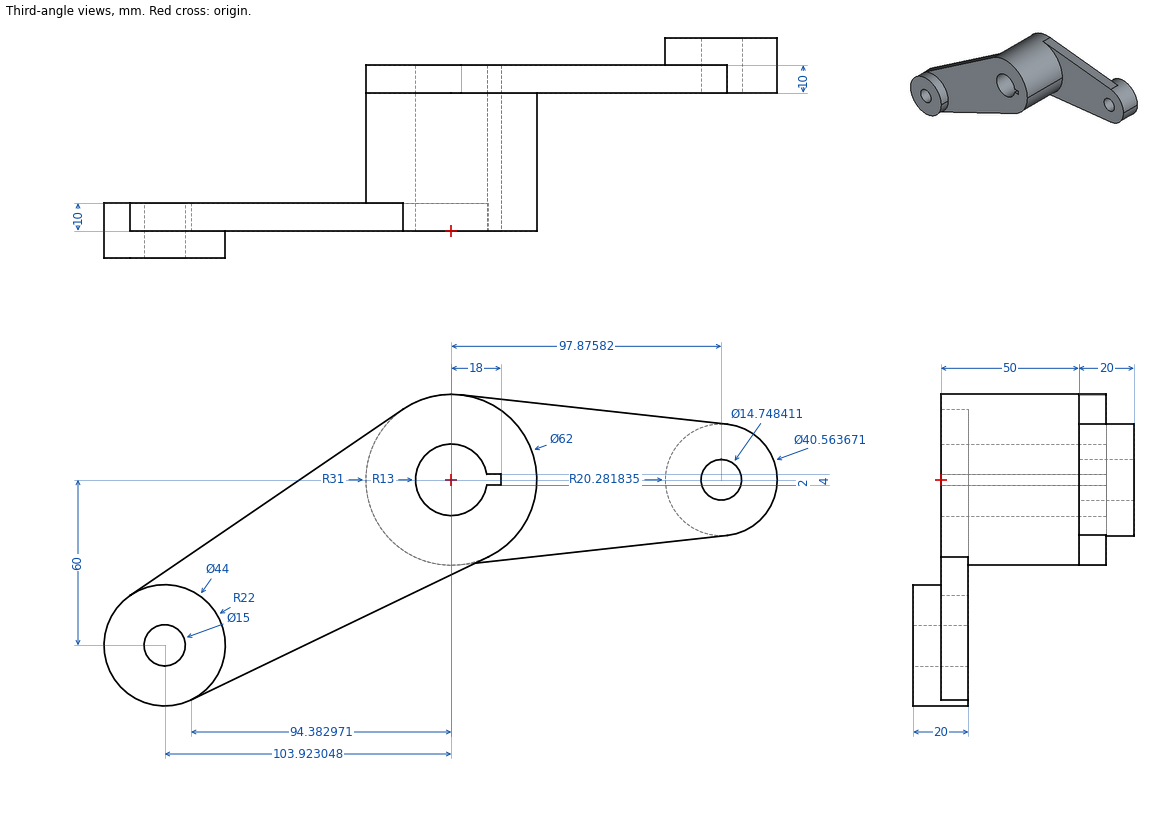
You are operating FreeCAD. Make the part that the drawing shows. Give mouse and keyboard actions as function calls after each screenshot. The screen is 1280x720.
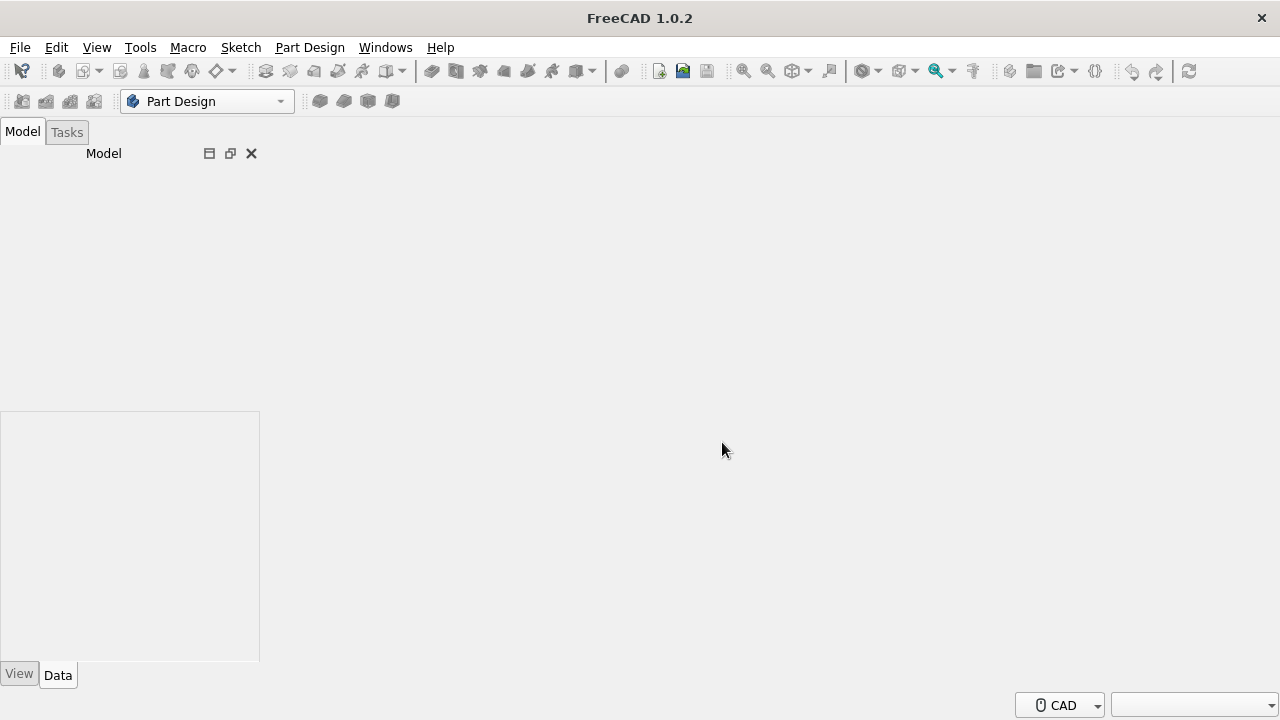
key(ctrl+n)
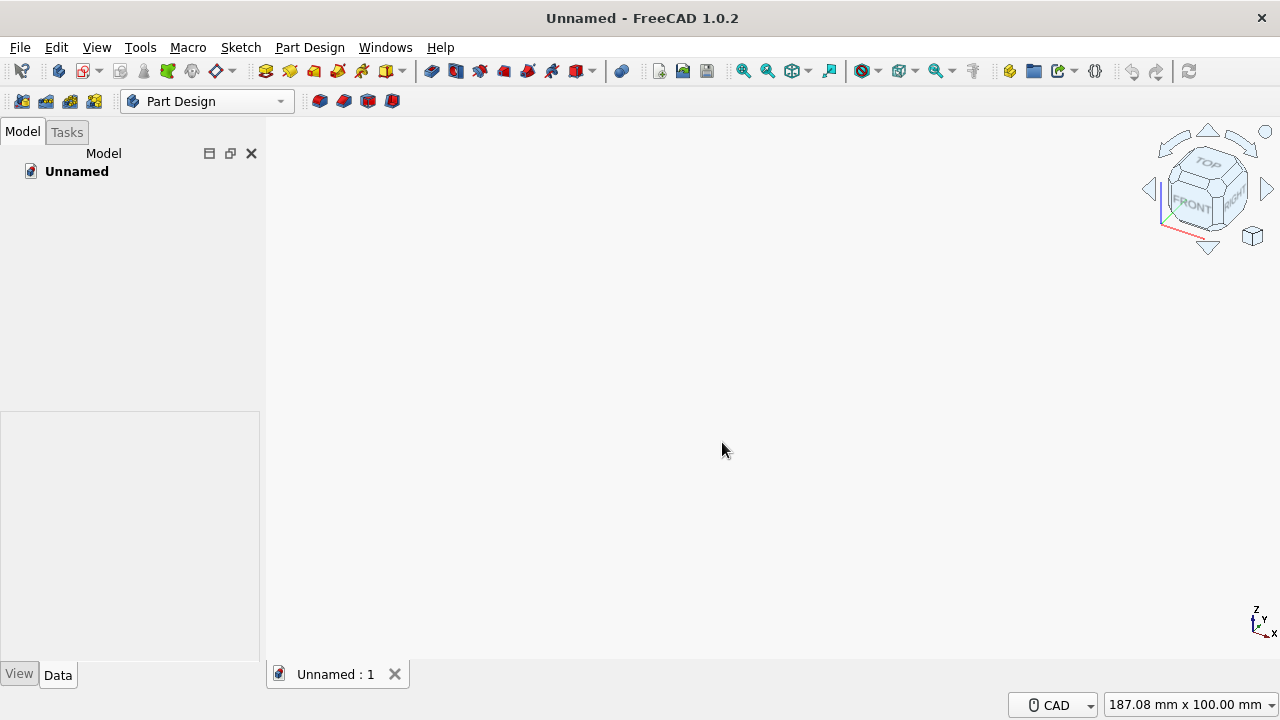
click(84, 72)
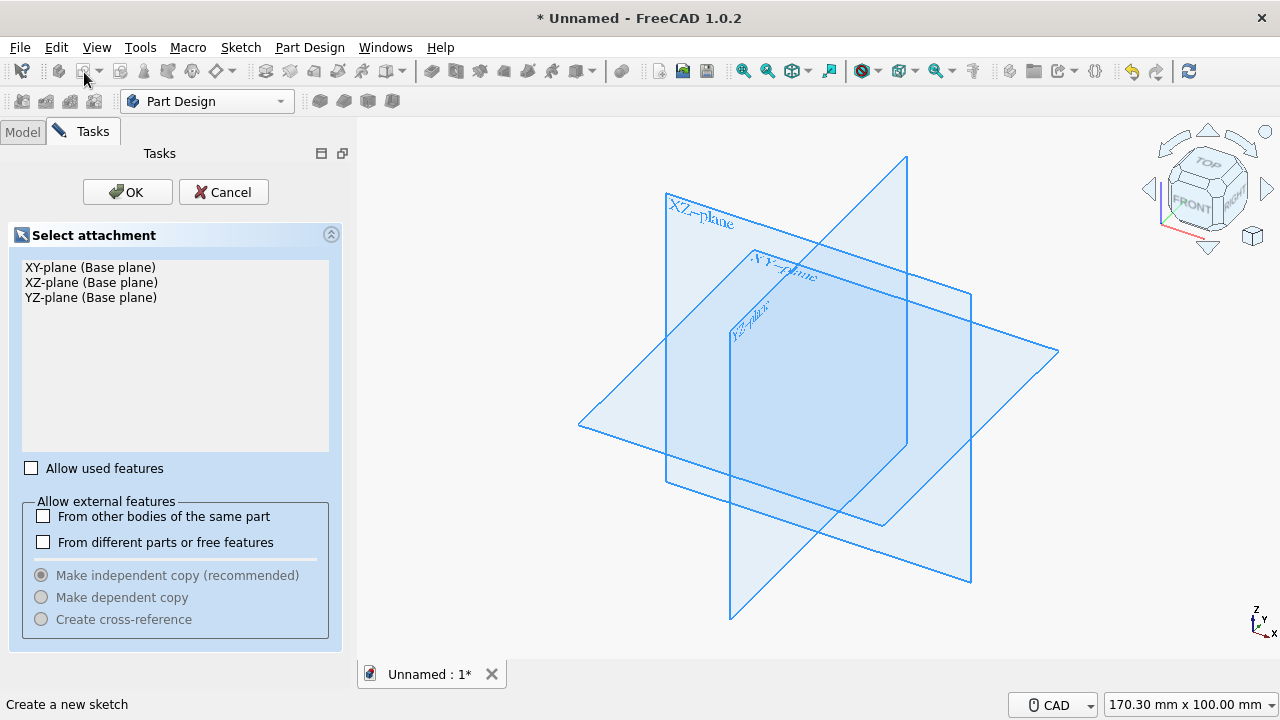
click(82, 282)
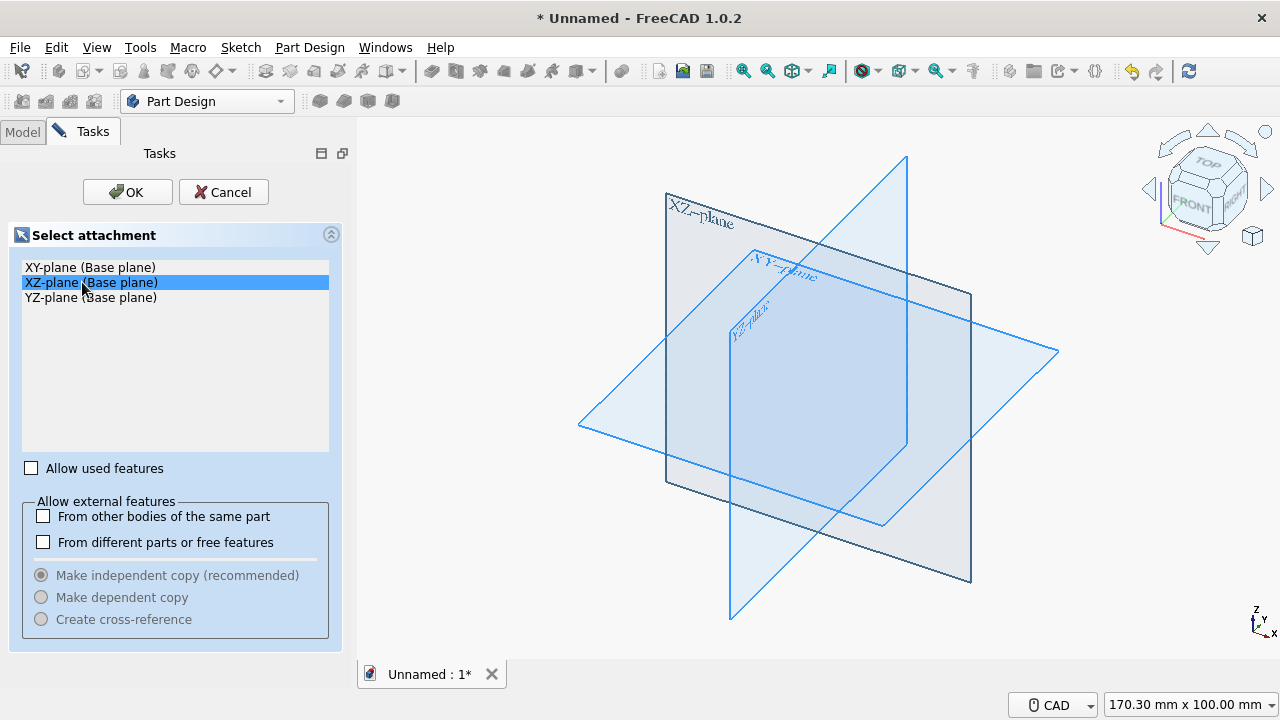
click(128, 192)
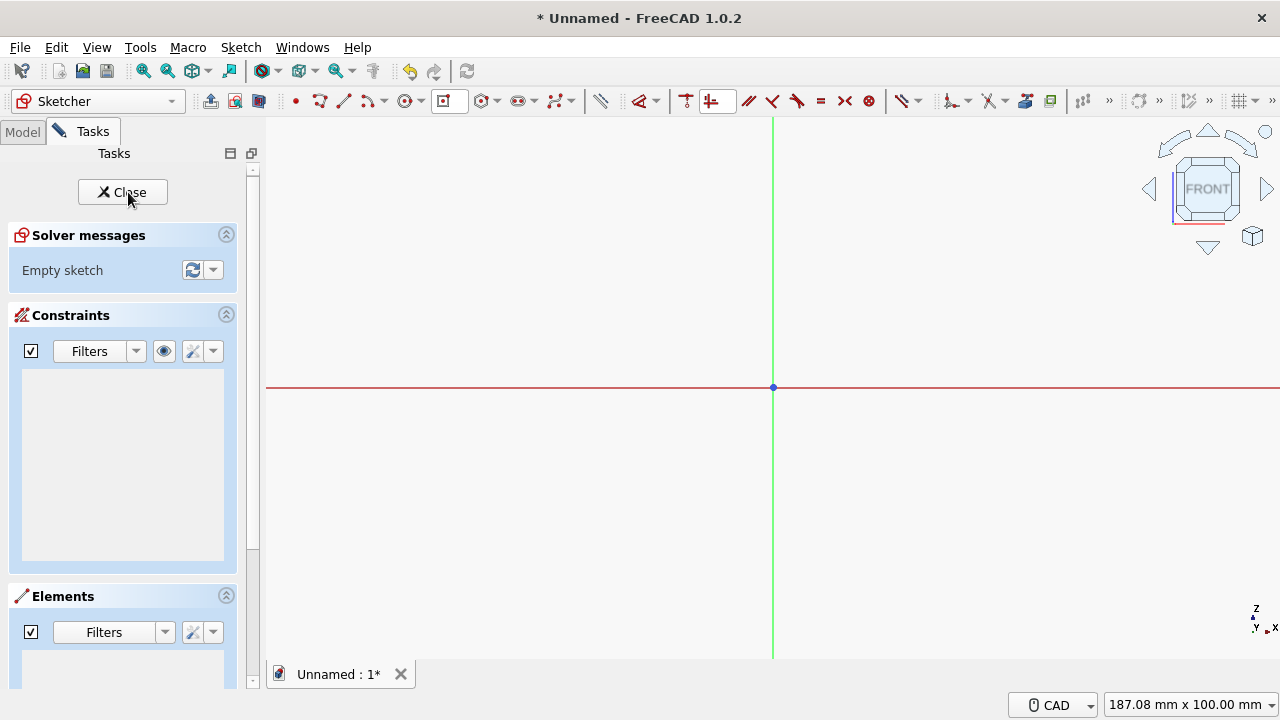
key(g)
key(m)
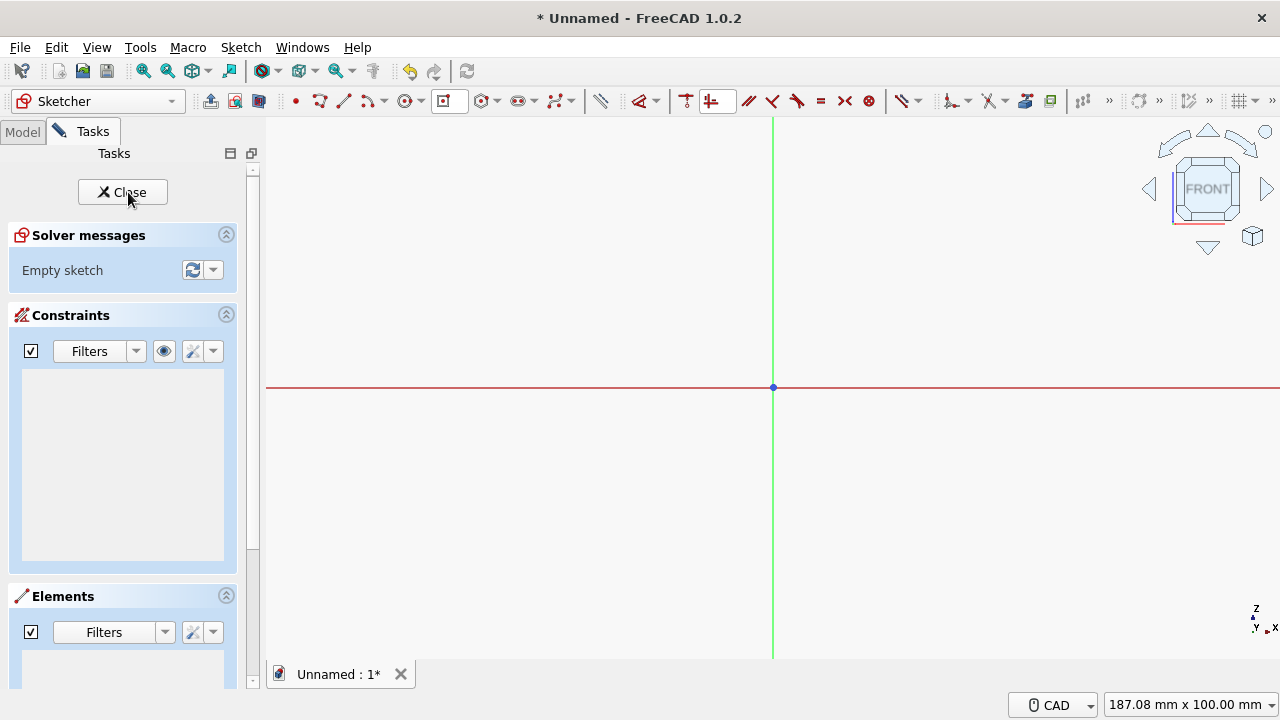
scroll(843, 399, up, 2)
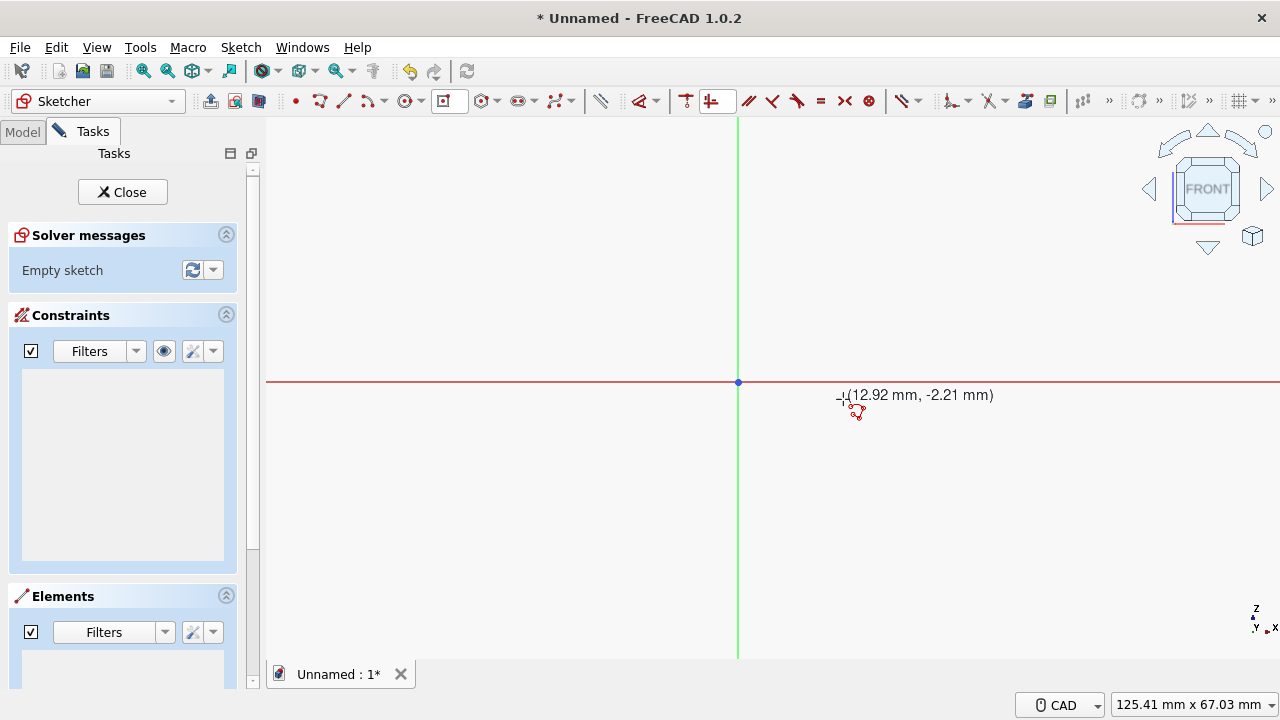
click(842, 399)
click(884, 399)
click(884, 366)
click(842, 366)
right_click(842, 366)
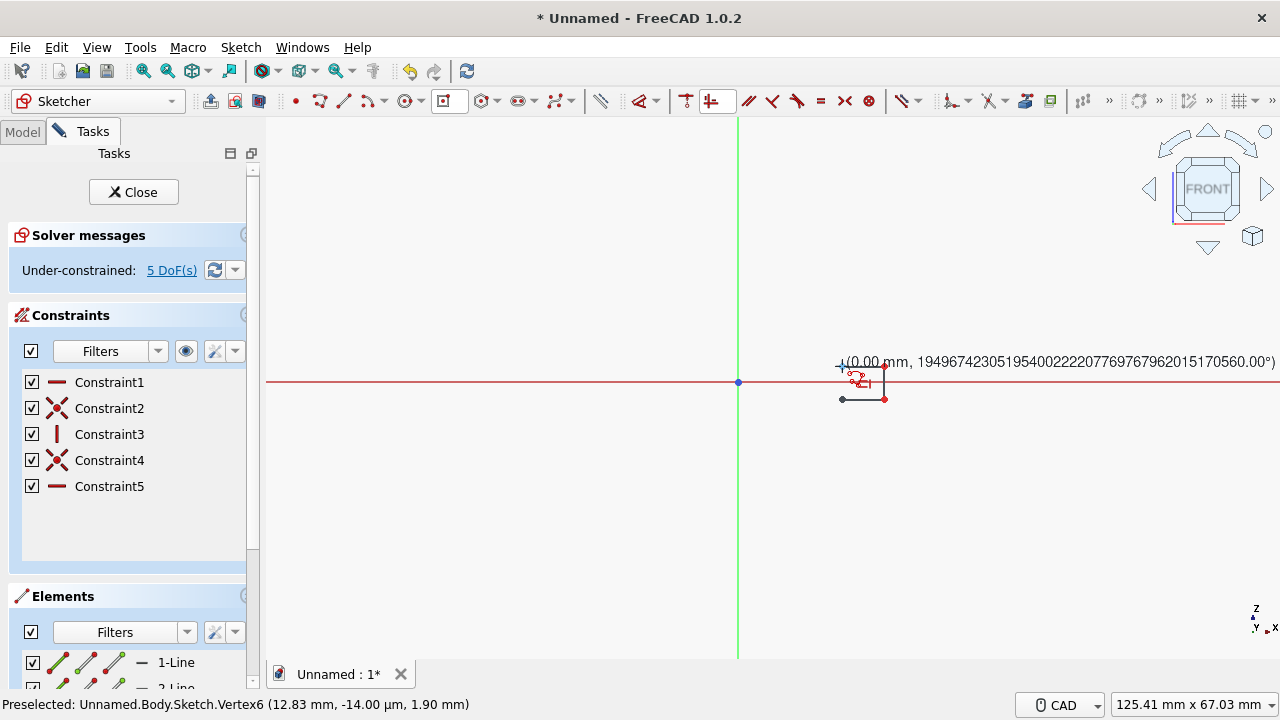
key(g)
key(3)
key(a)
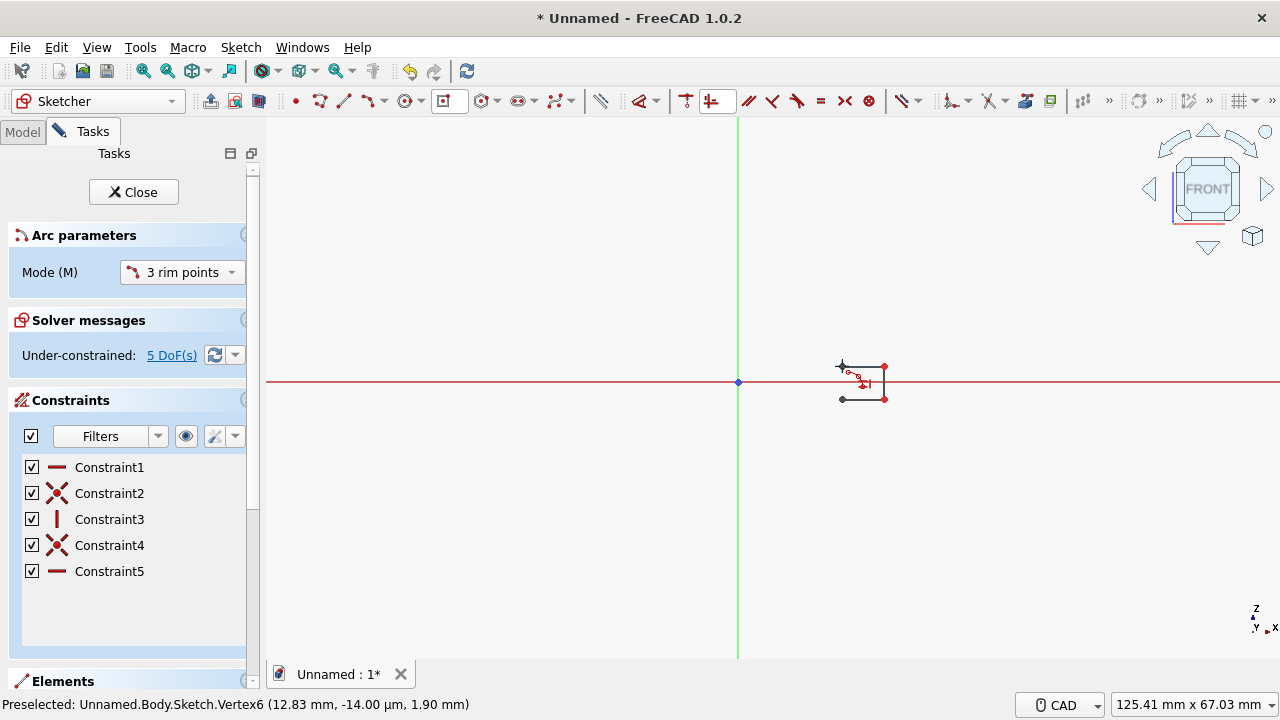
click(842, 367)
click(842, 400)
click(651, 323)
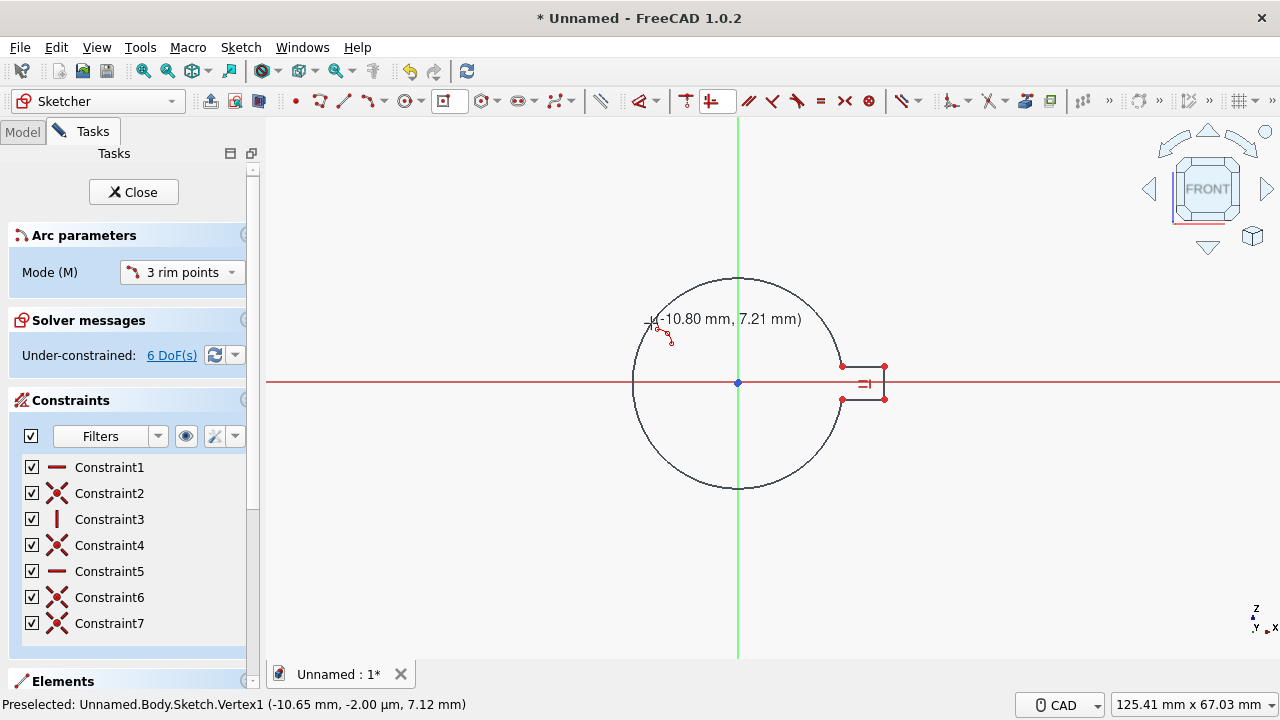
click(406, 102)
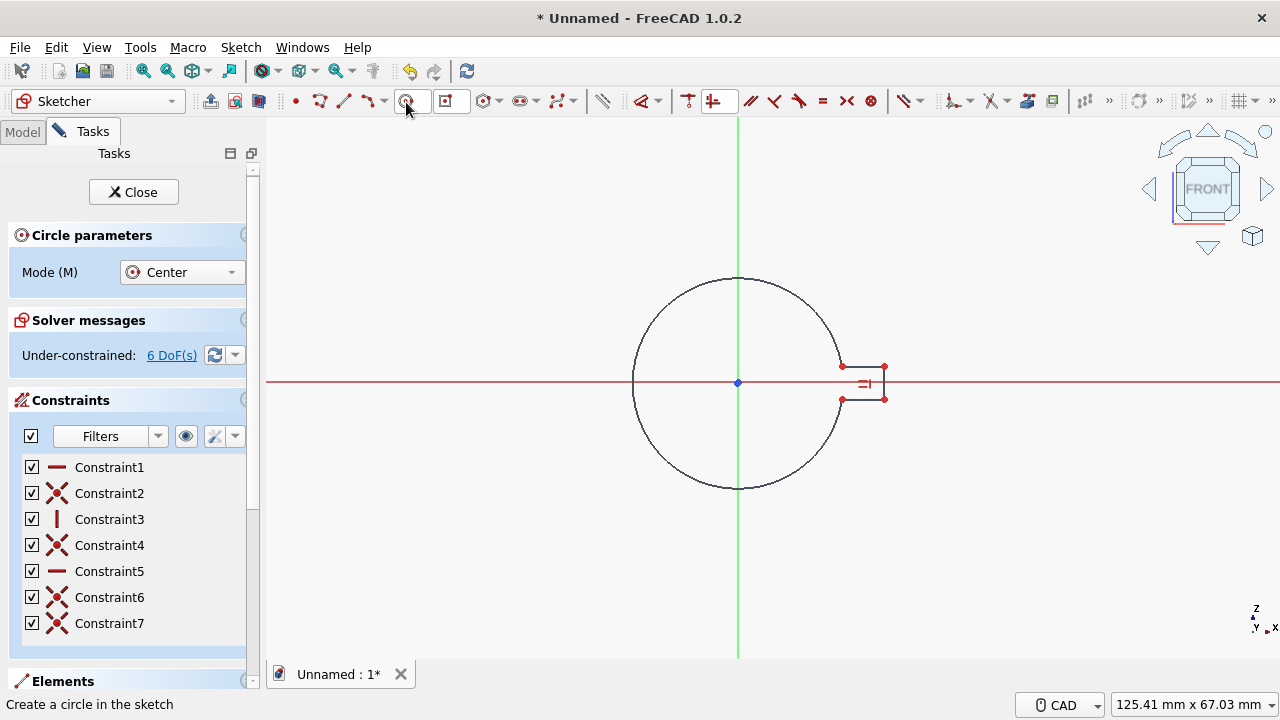
click(738, 382)
move(916, 205)